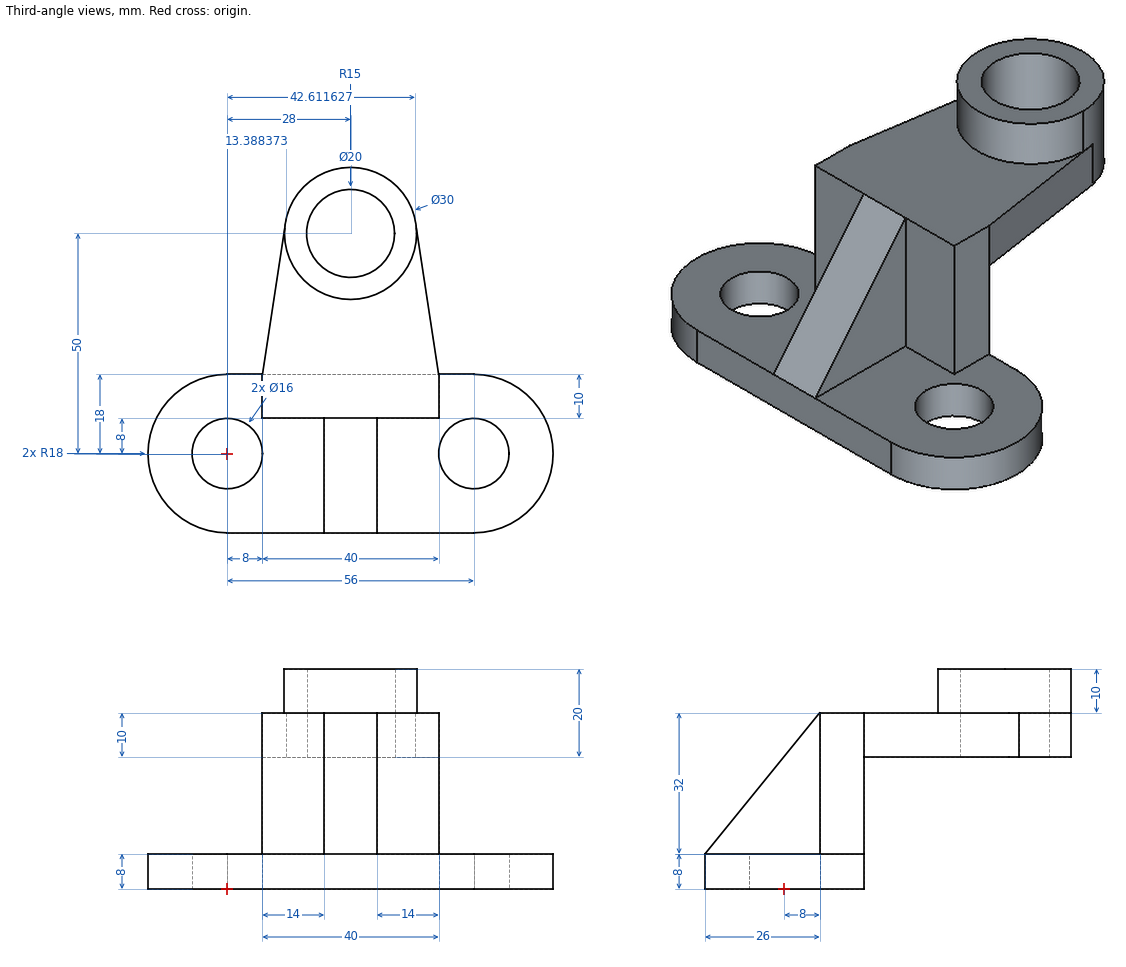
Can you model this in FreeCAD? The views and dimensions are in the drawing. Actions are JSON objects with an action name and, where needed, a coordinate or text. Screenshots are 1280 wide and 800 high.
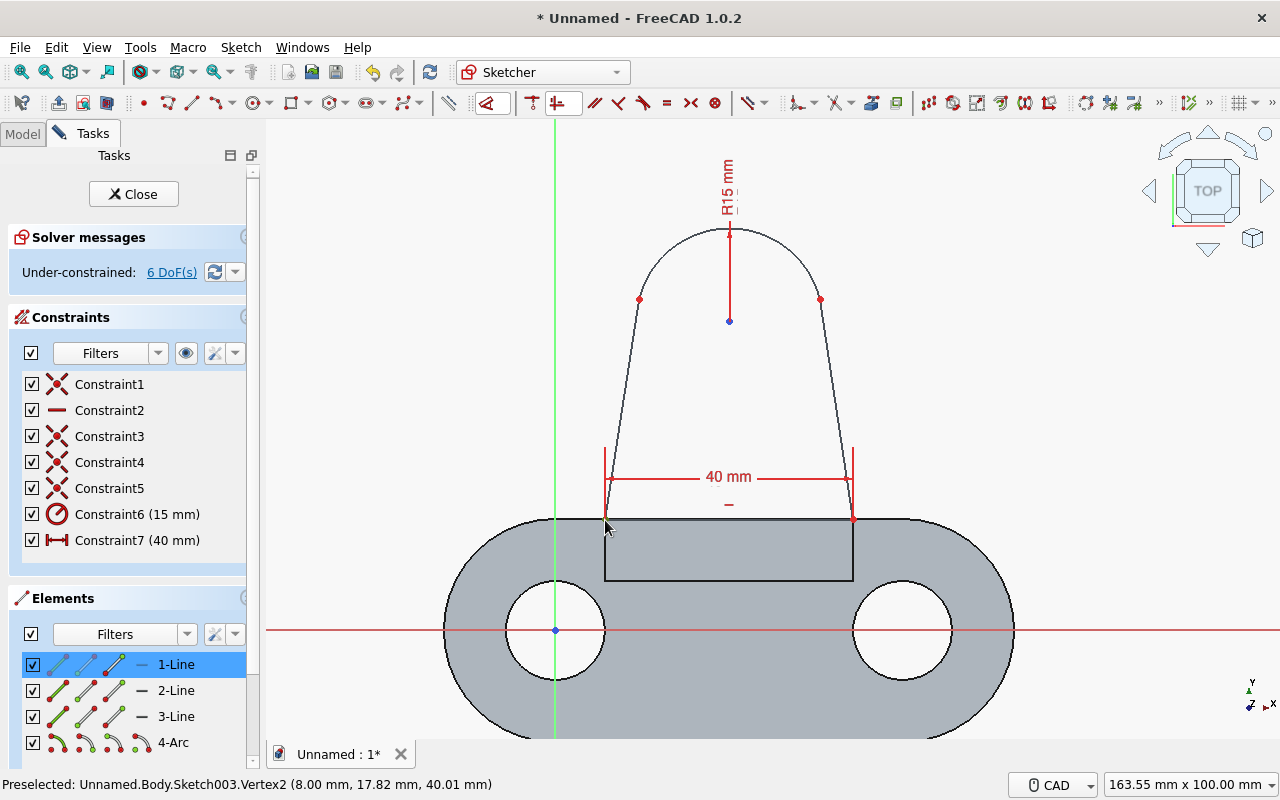
{"action": "key", "text": "l"}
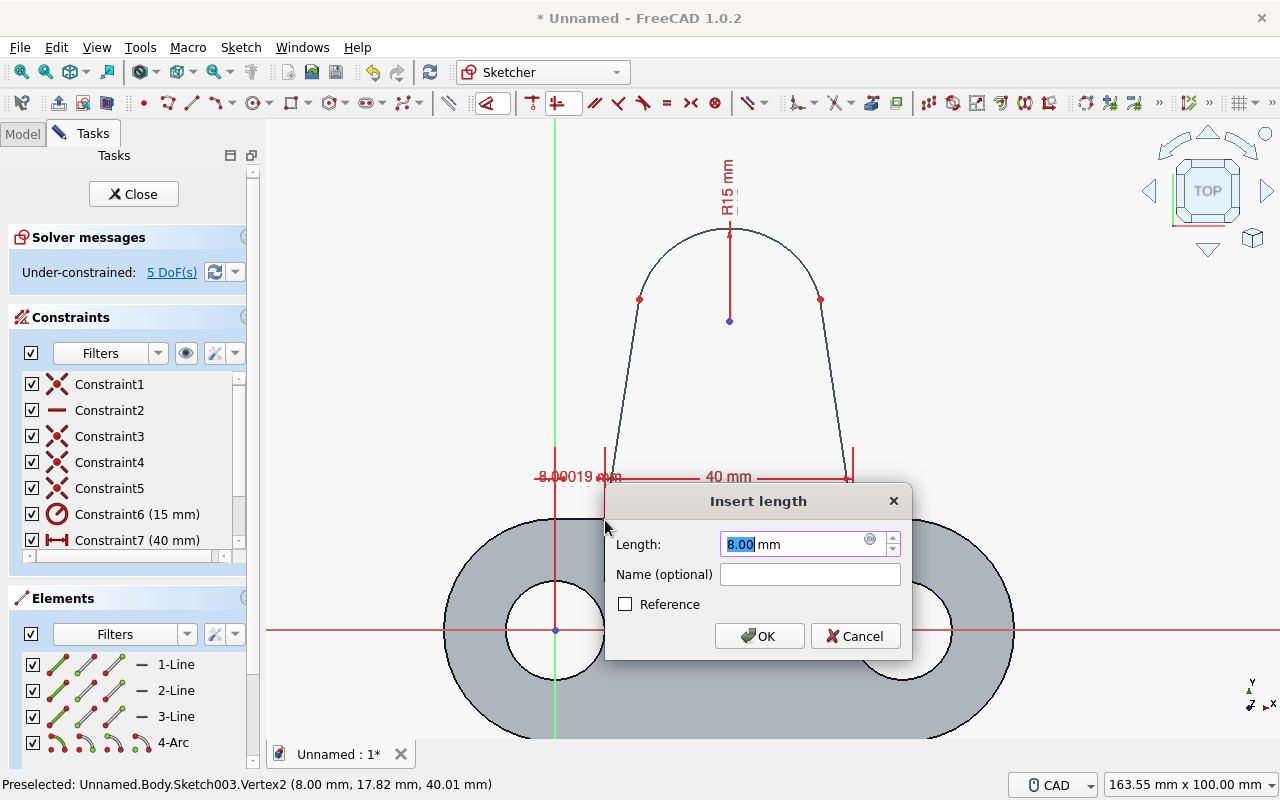
{"action": "type", "text": "8"}
{"action": "key", "text": "Return"}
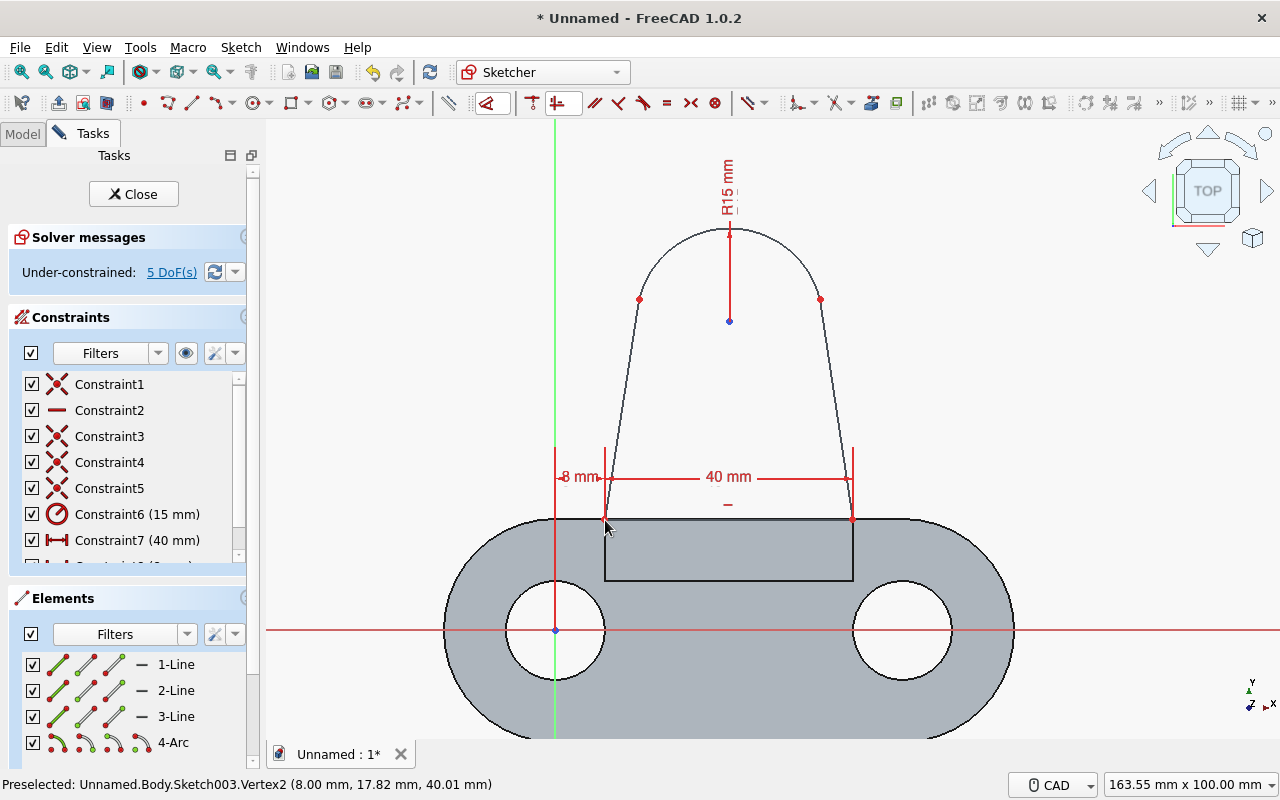
{"action": "left_click", "coordinate": [605, 520]}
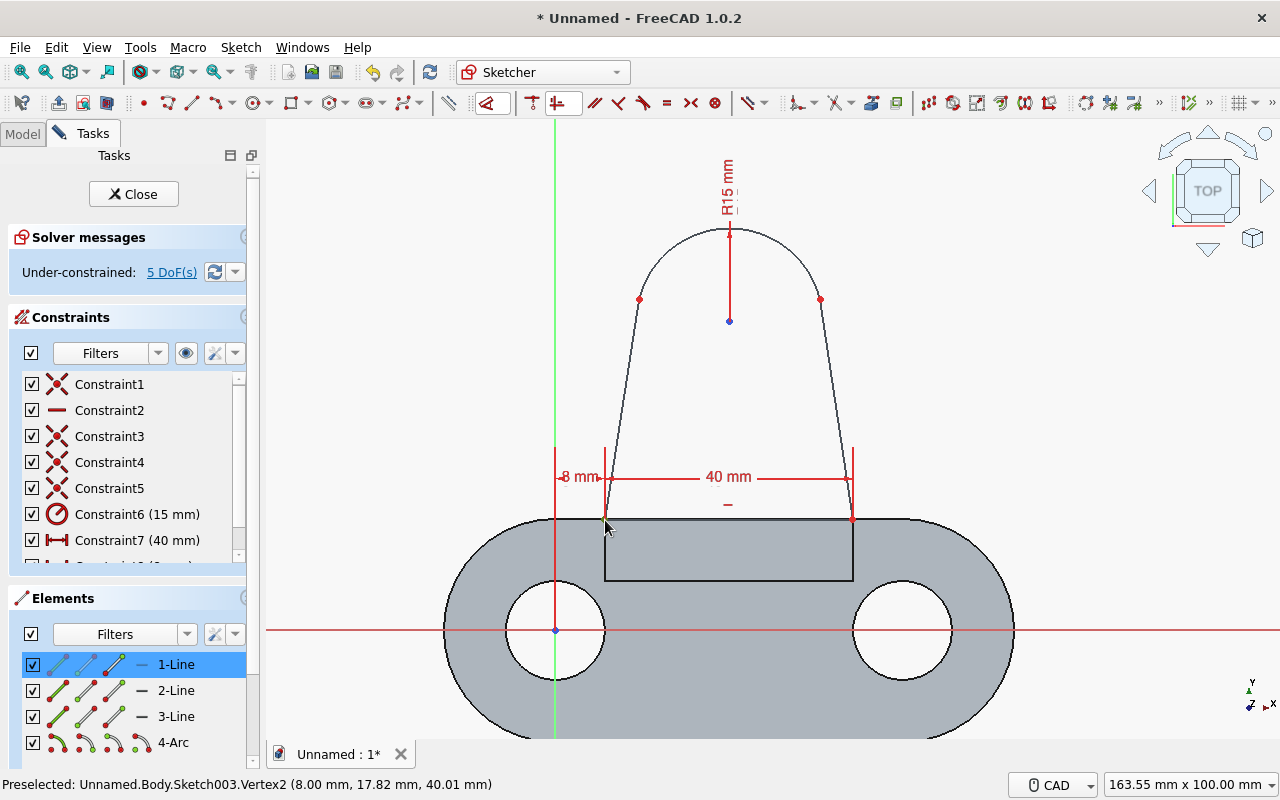
{"action": "left_click", "coordinate": [504, 104]}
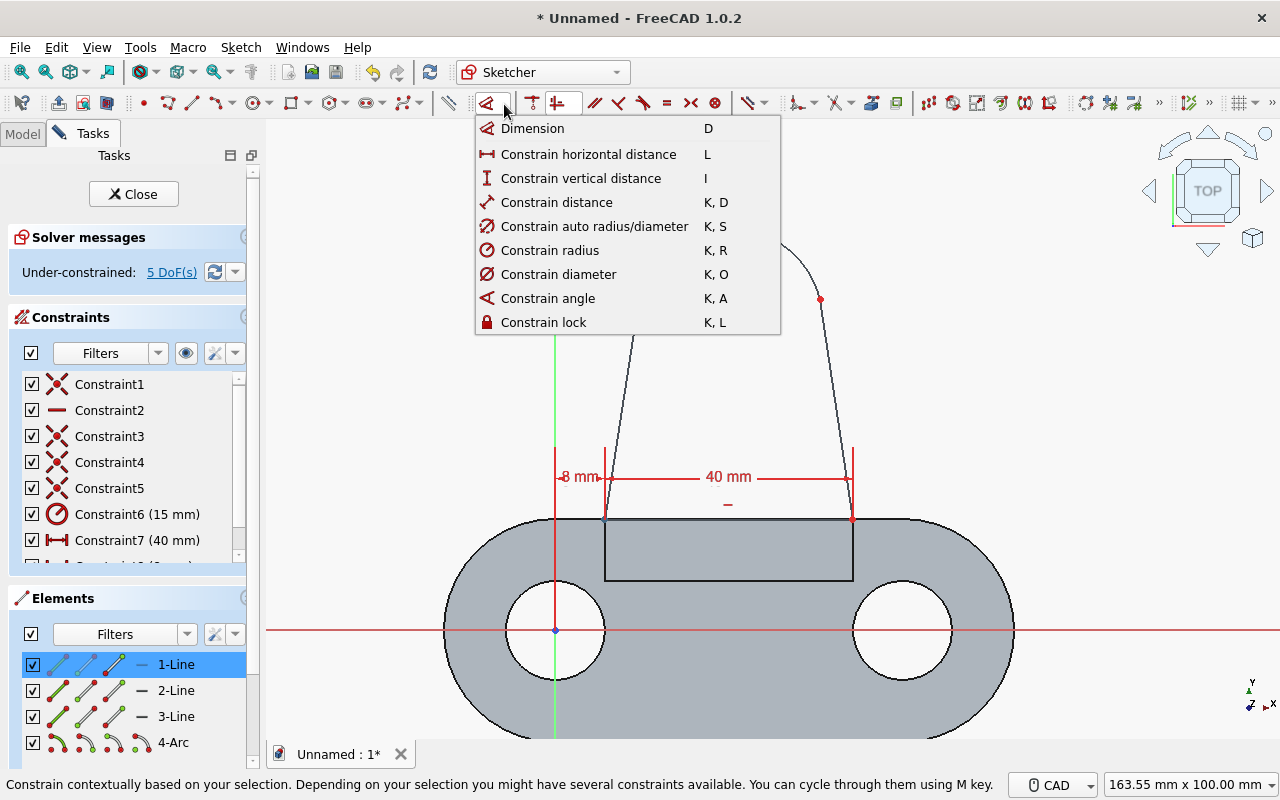
{"action": "left_click", "coordinate": [628, 178]}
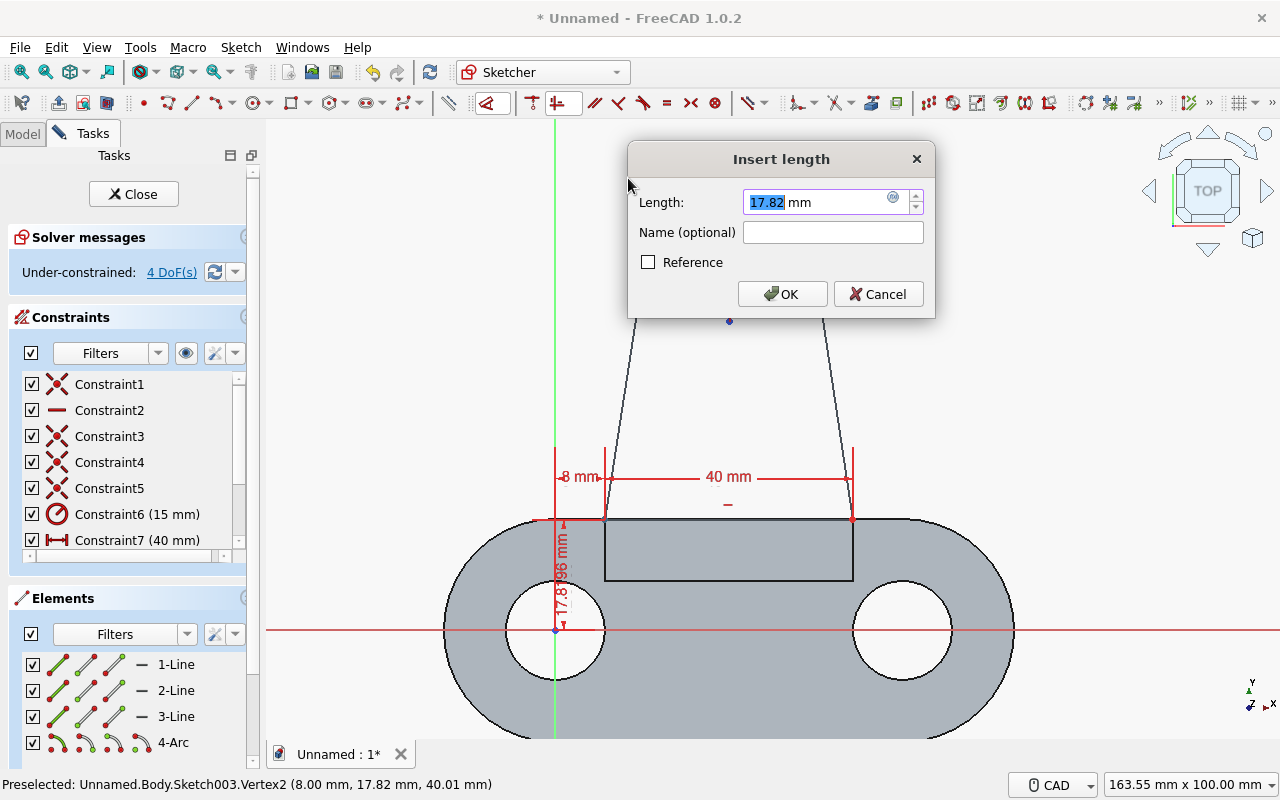
{"action": "type", "text": "18"}
{"action": "key", "text": "Return"}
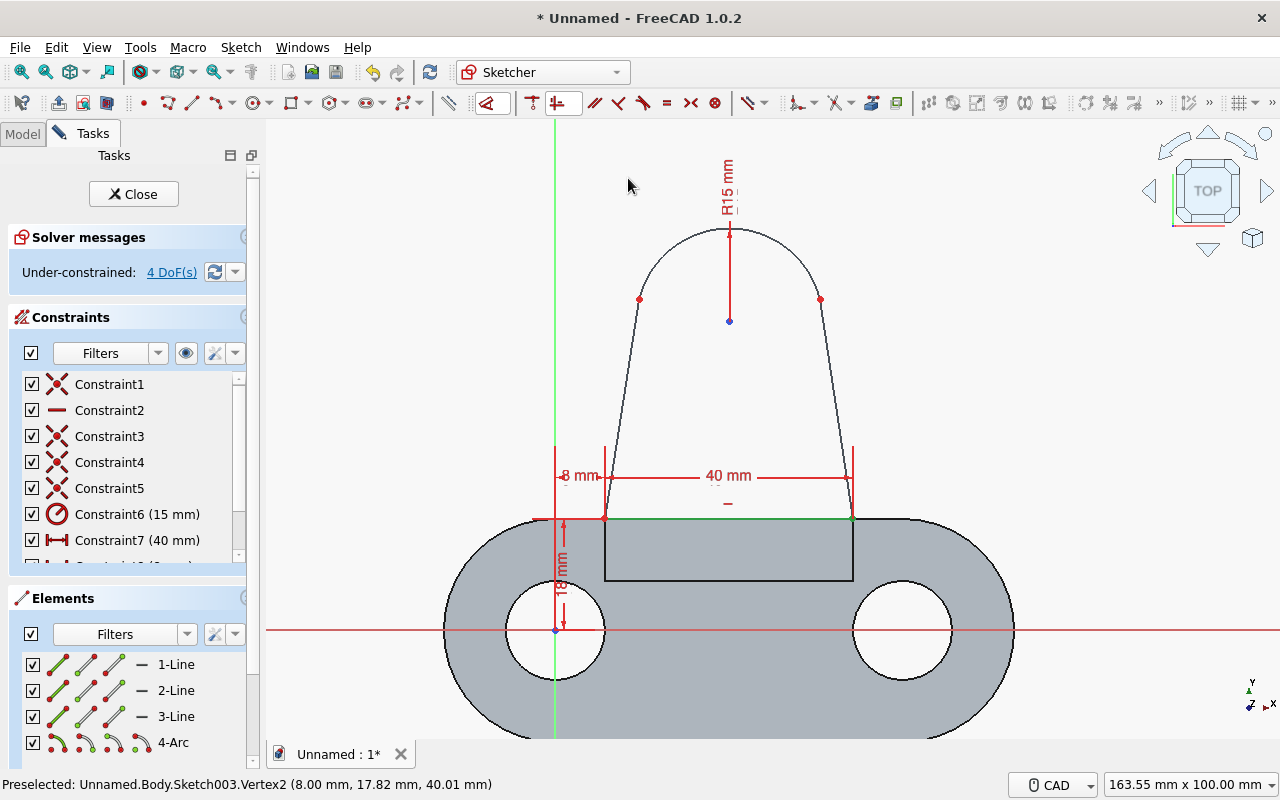
{"action": "left_click", "coordinate": [730, 322]}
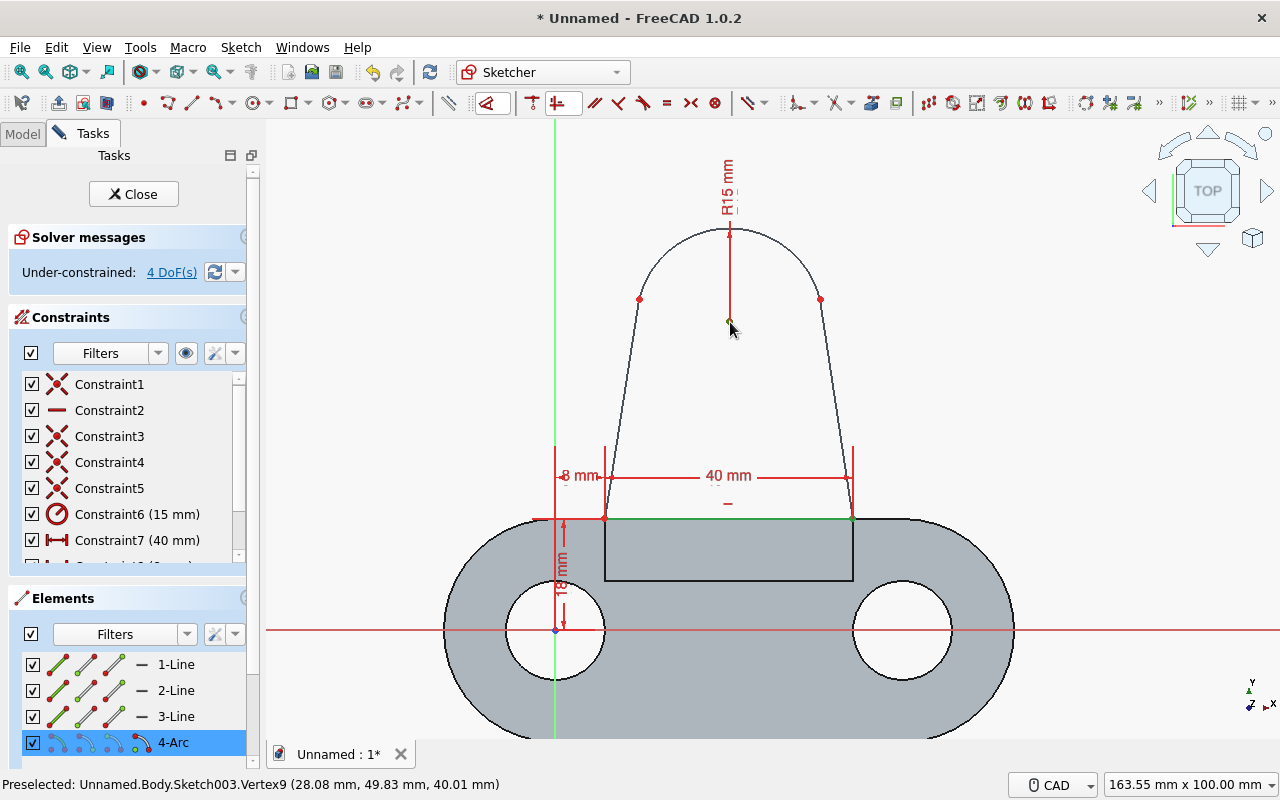
{"action": "left_click", "coordinate": [504, 104]}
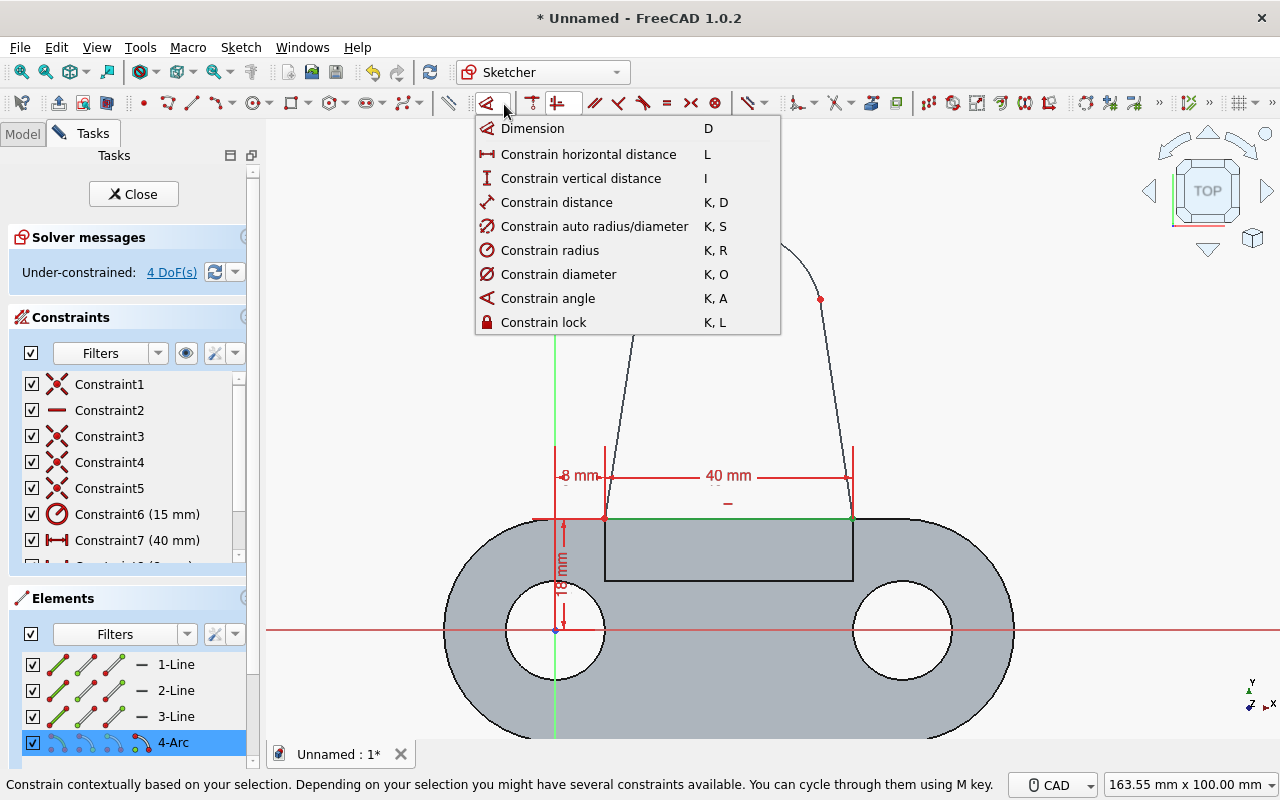
{"action": "left_click", "coordinate": [628, 154]}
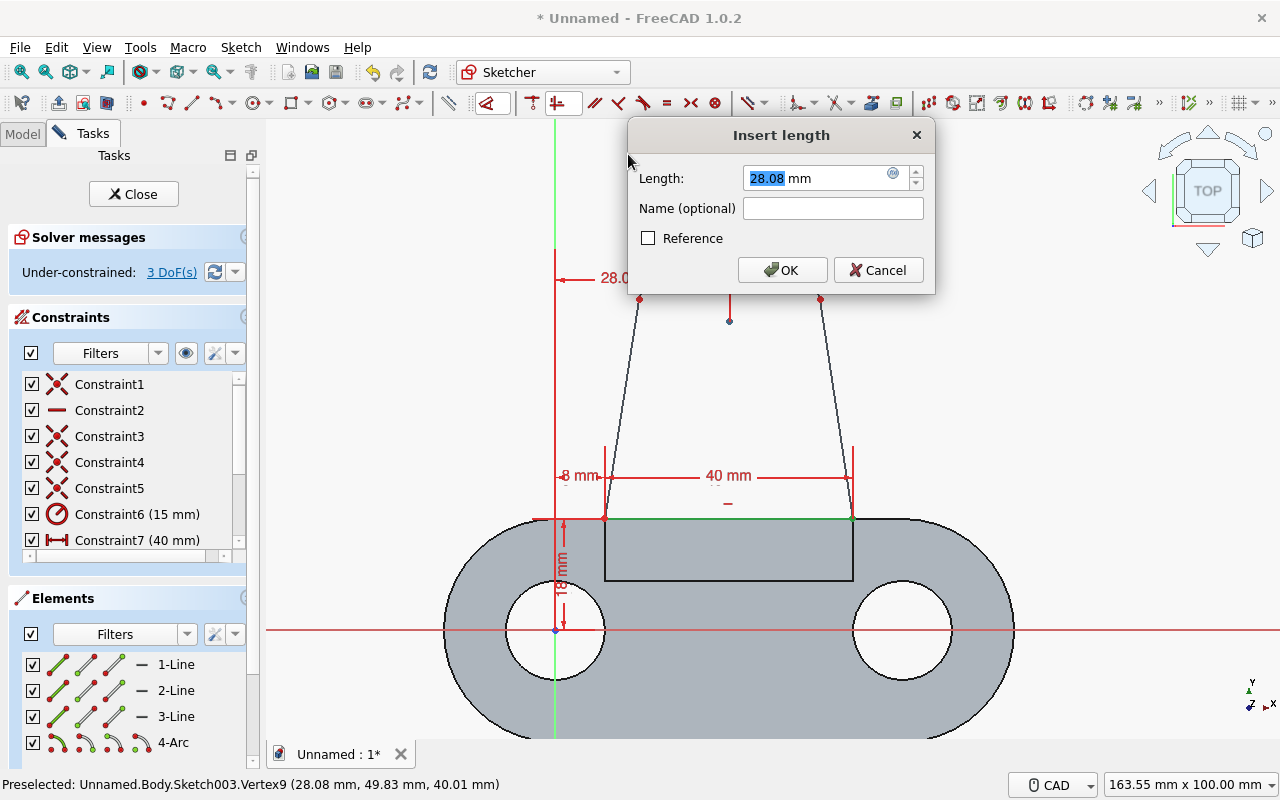
{"action": "type", "text": "28"}
{"action": "key", "text": "Return"}